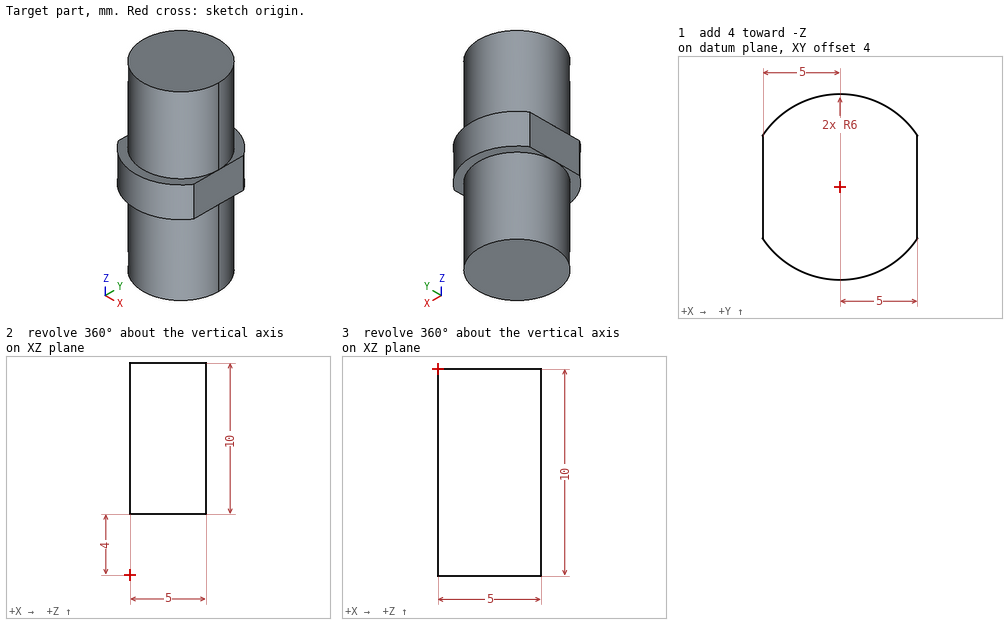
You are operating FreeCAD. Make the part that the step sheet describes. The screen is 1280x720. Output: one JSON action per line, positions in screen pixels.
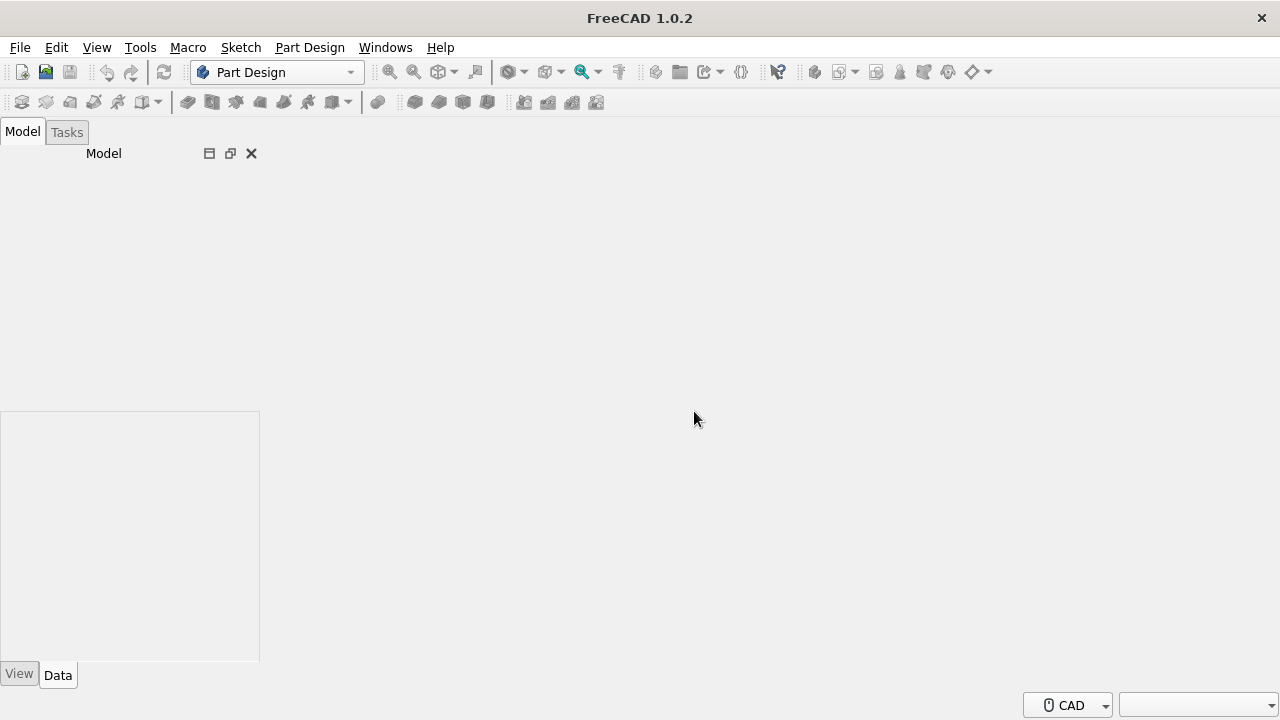
{"action": "left_click", "coordinate": [22, 72]}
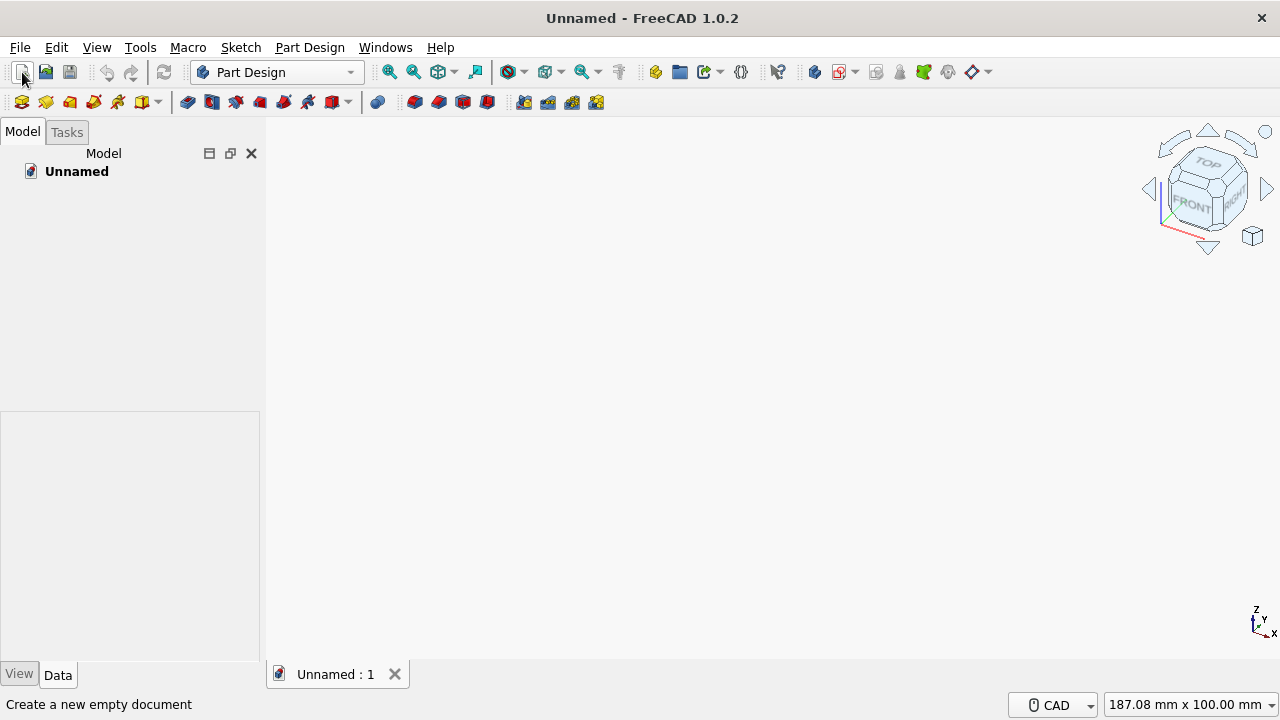
{"action": "left_click", "coordinate": [816, 72]}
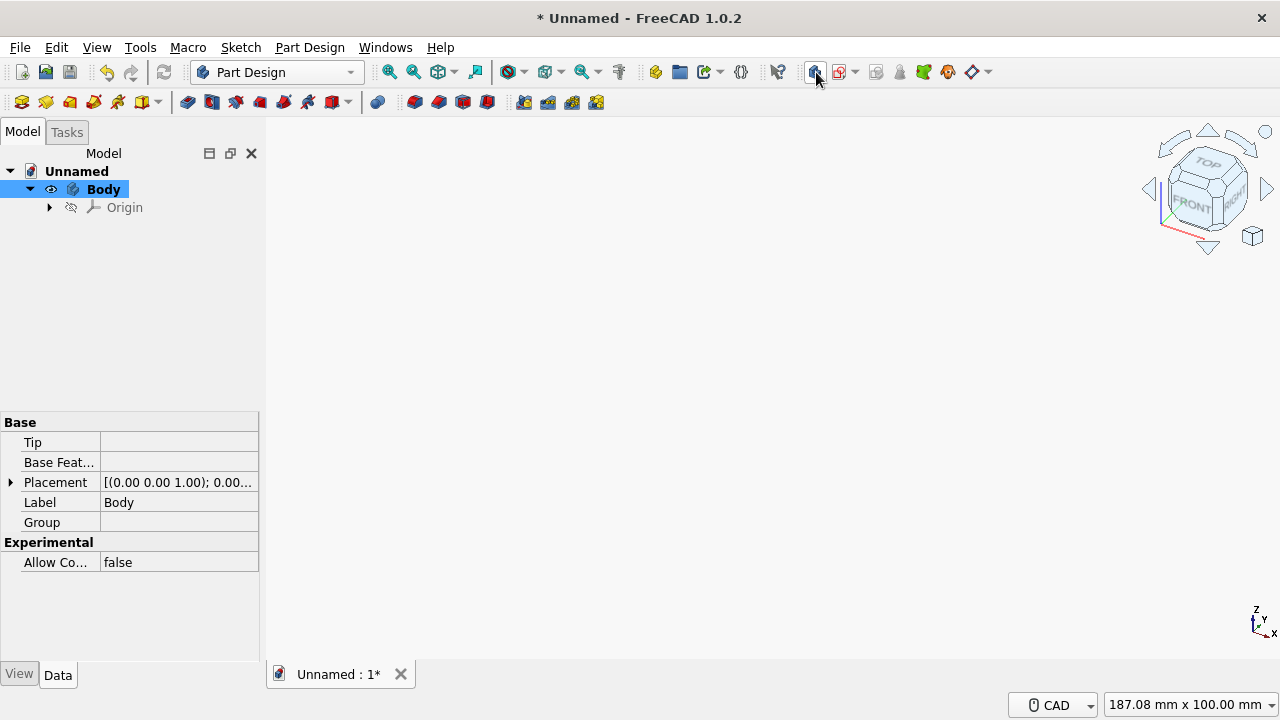
{"action": "left_click", "coordinate": [50, 207]}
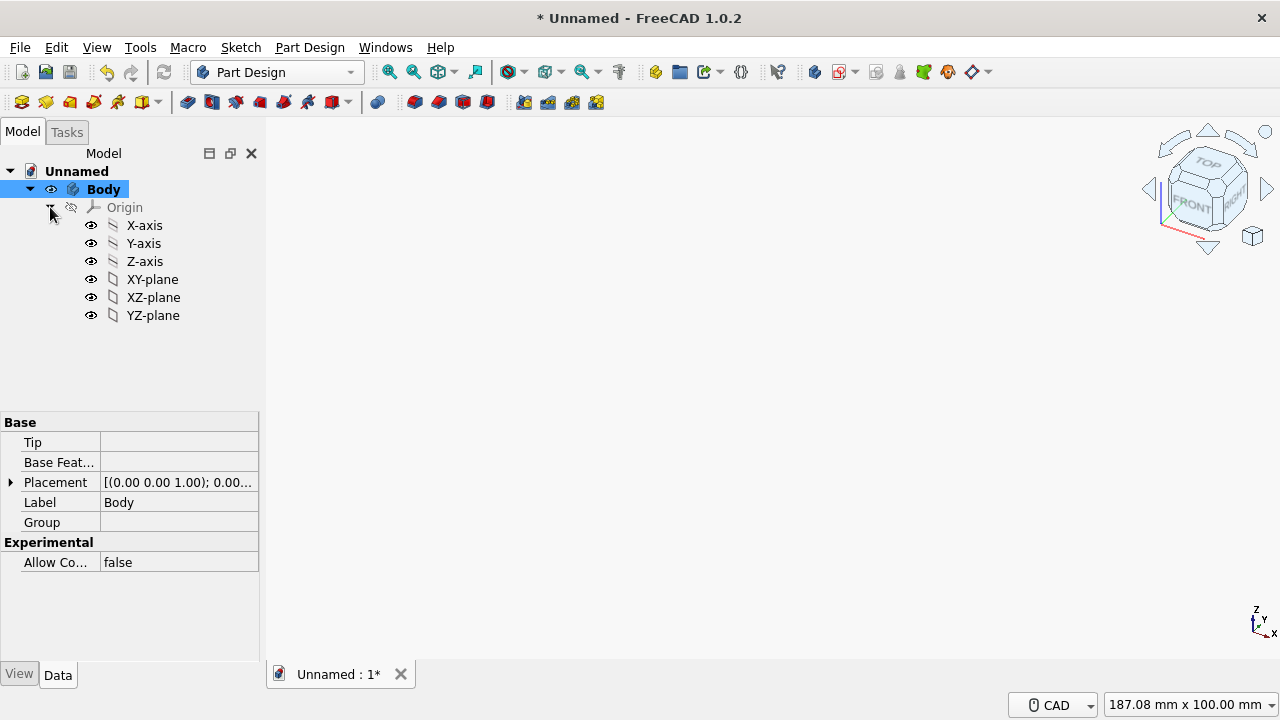
{"action": "left_click", "coordinate": [136, 279]}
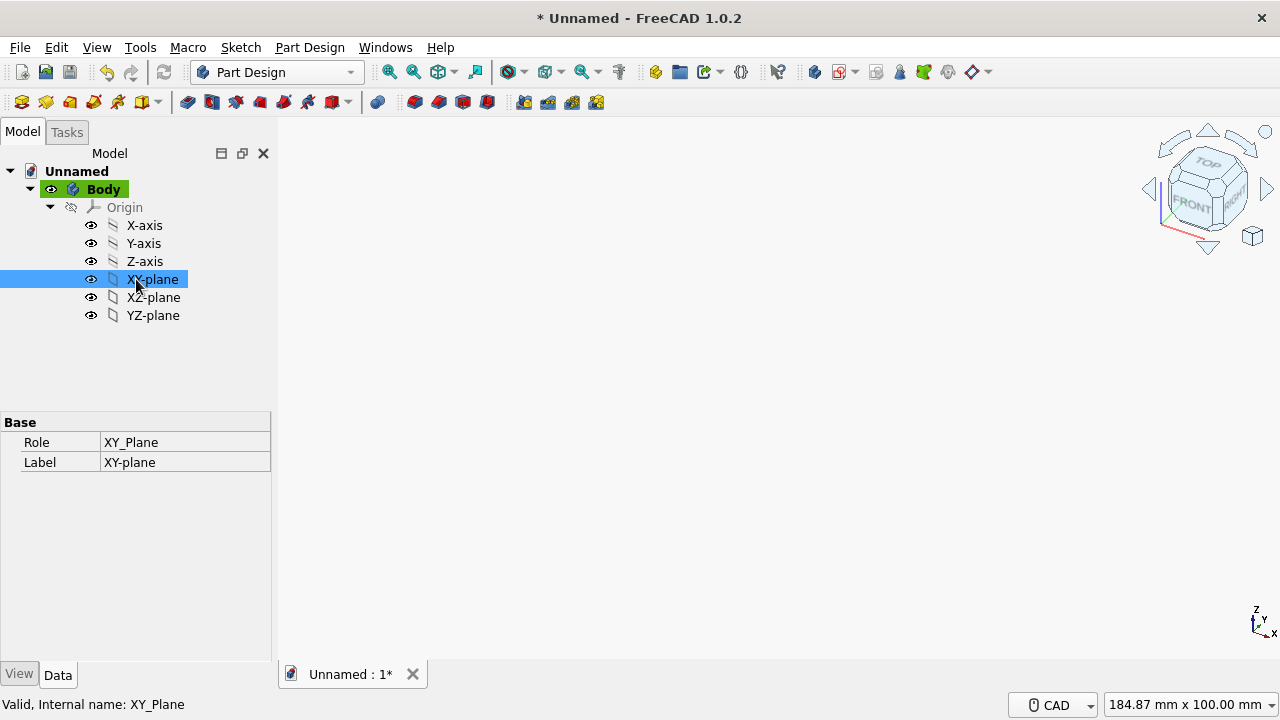
{"action": "left_click", "coordinate": [972, 72]}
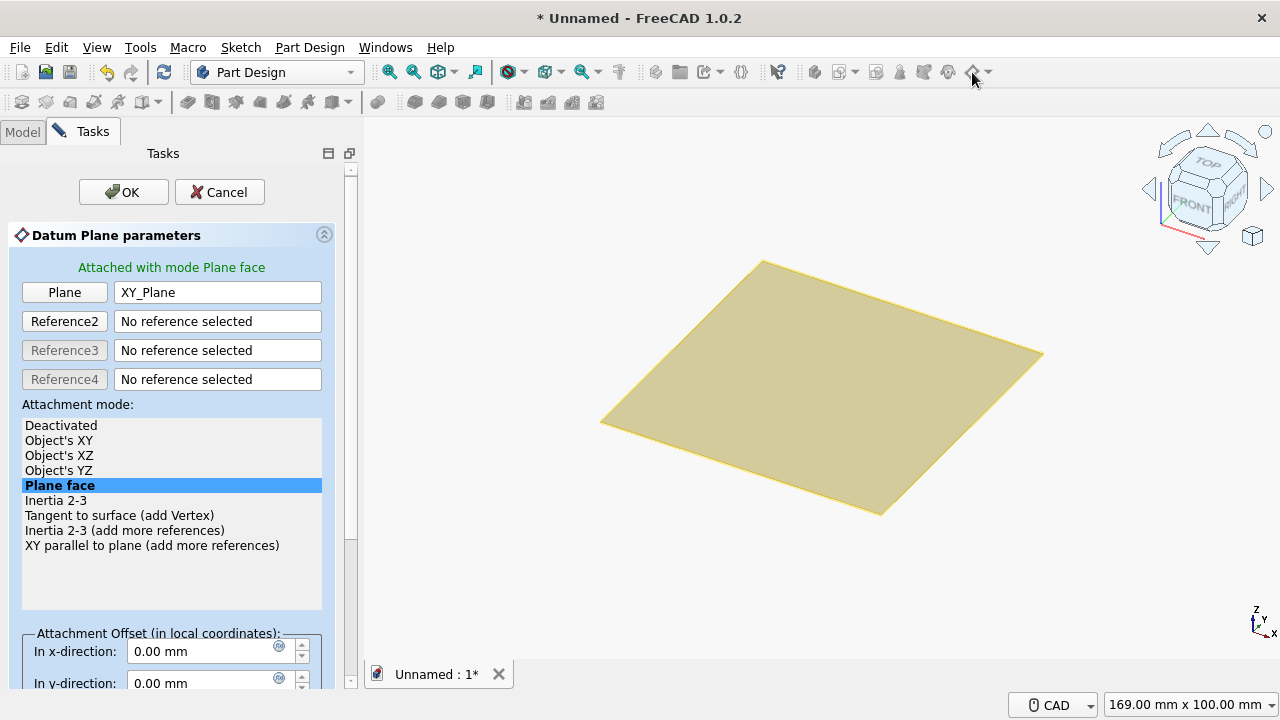
{"action": "scroll", "coordinate": [351, 426], "scroll_direction": "down", "scroll_amount": 2}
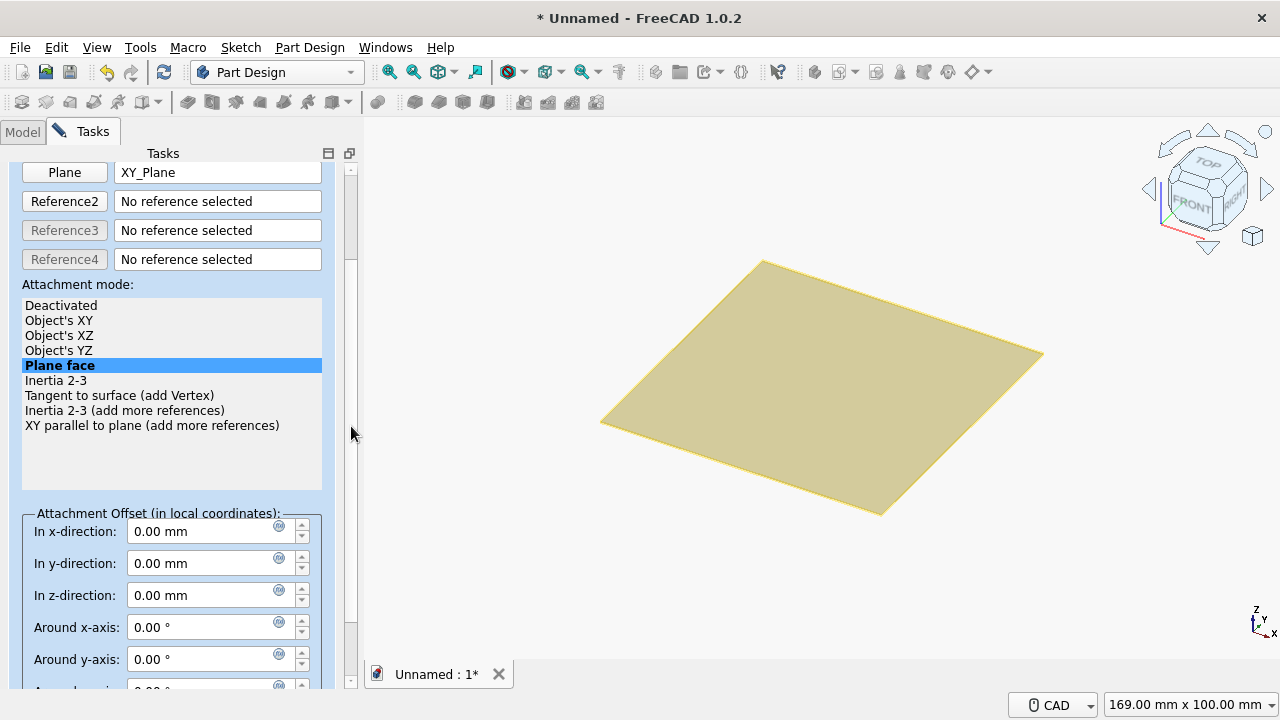
{"action": "triple_click", "coordinate": [210, 595]}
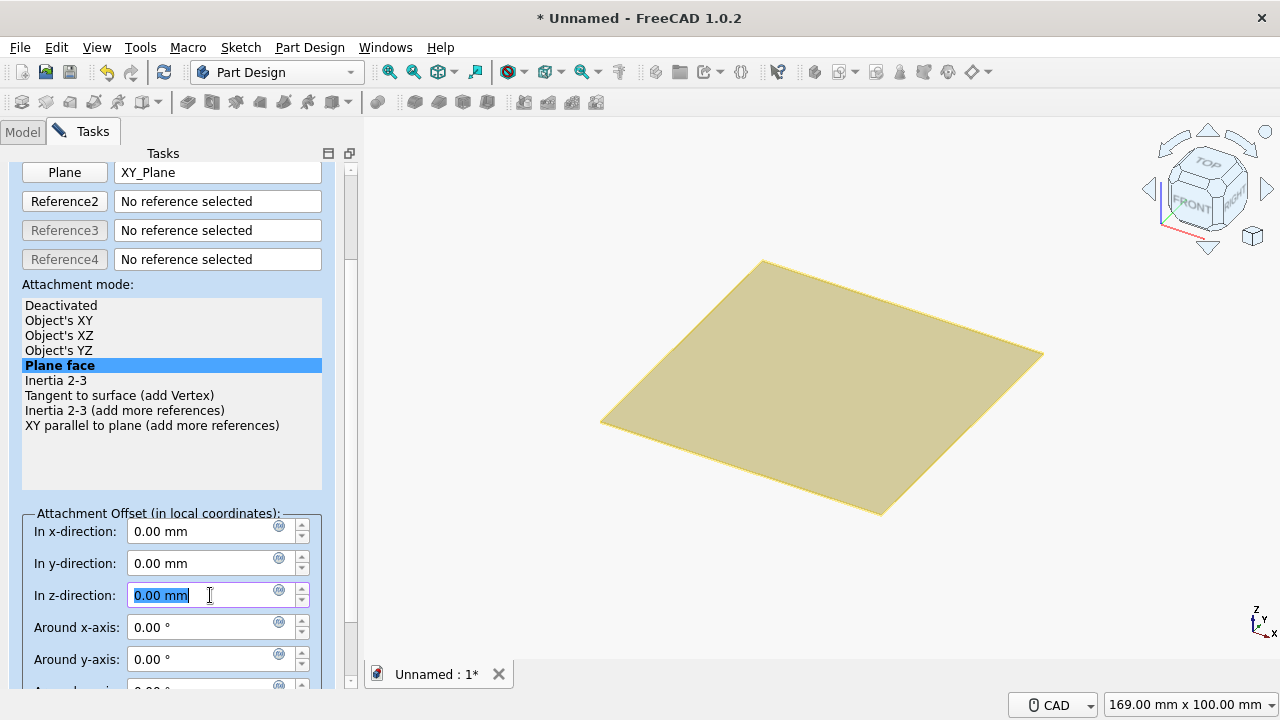
{"action": "type", "text": "4"}
{"action": "key", "text": "Tab"}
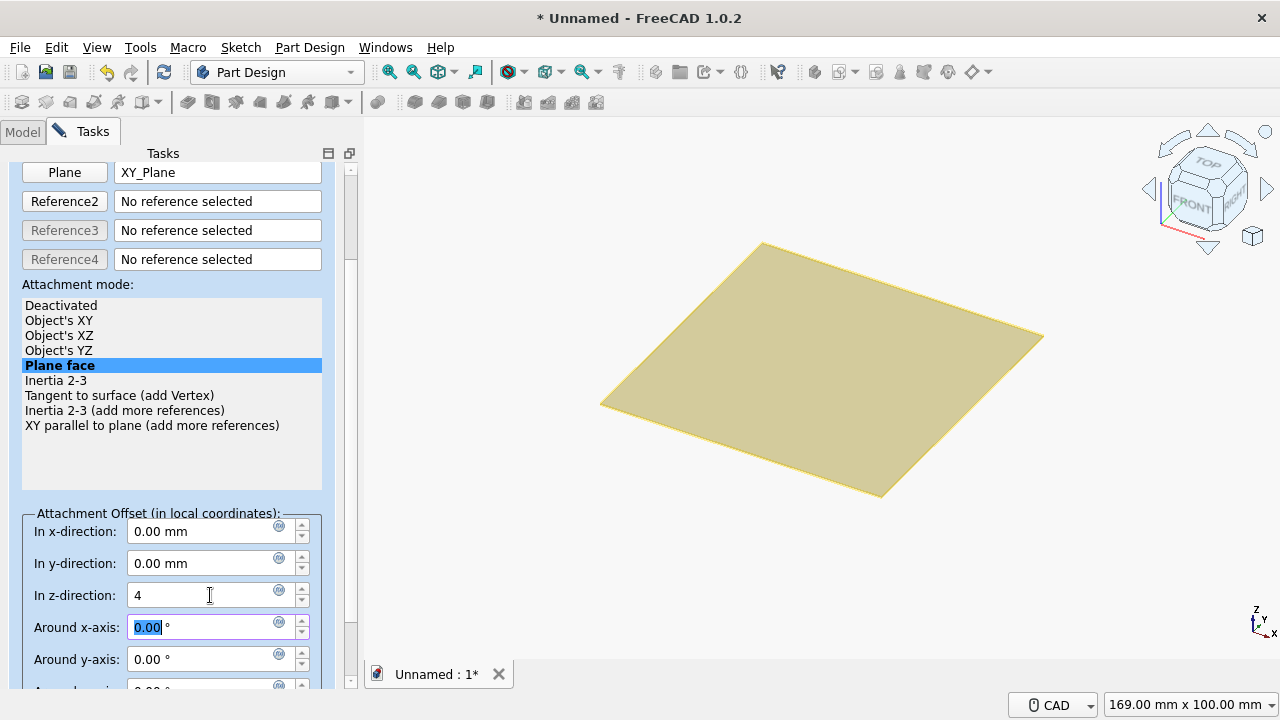
{"action": "scroll", "coordinate": [351, 426], "scroll_direction": "up", "scroll_amount": 3}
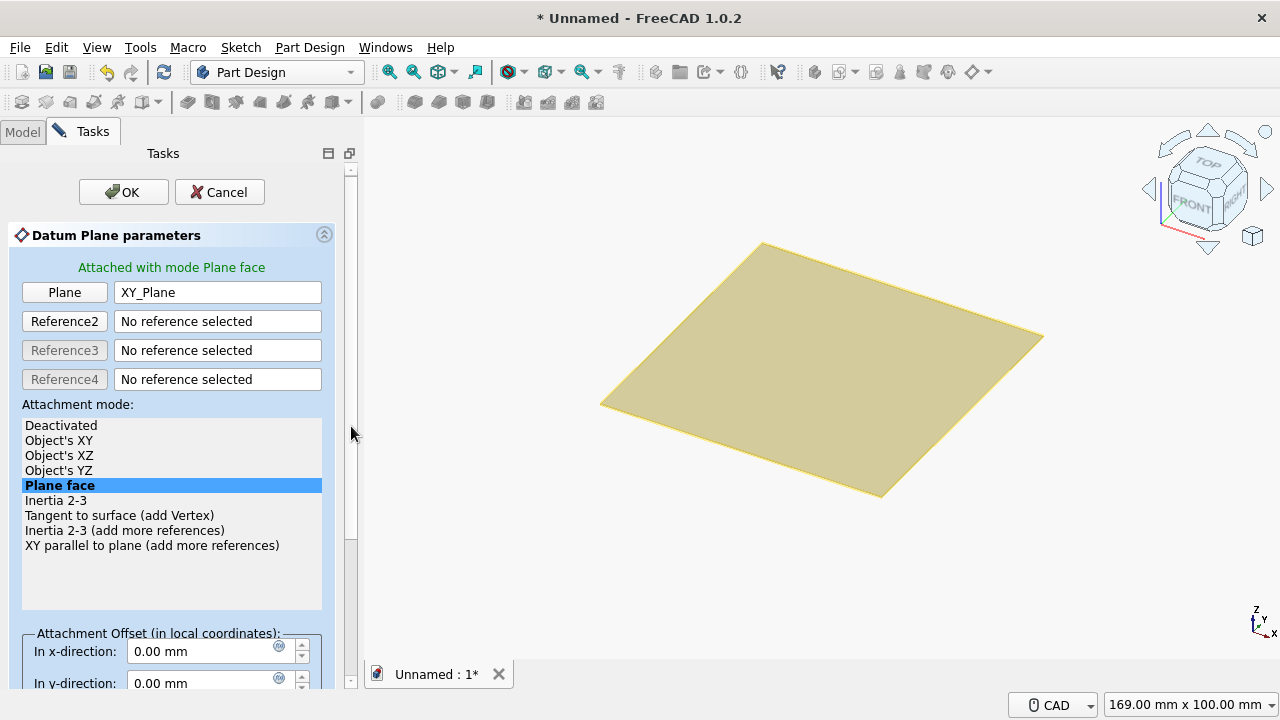
{"action": "left_click", "coordinate": [124, 192]}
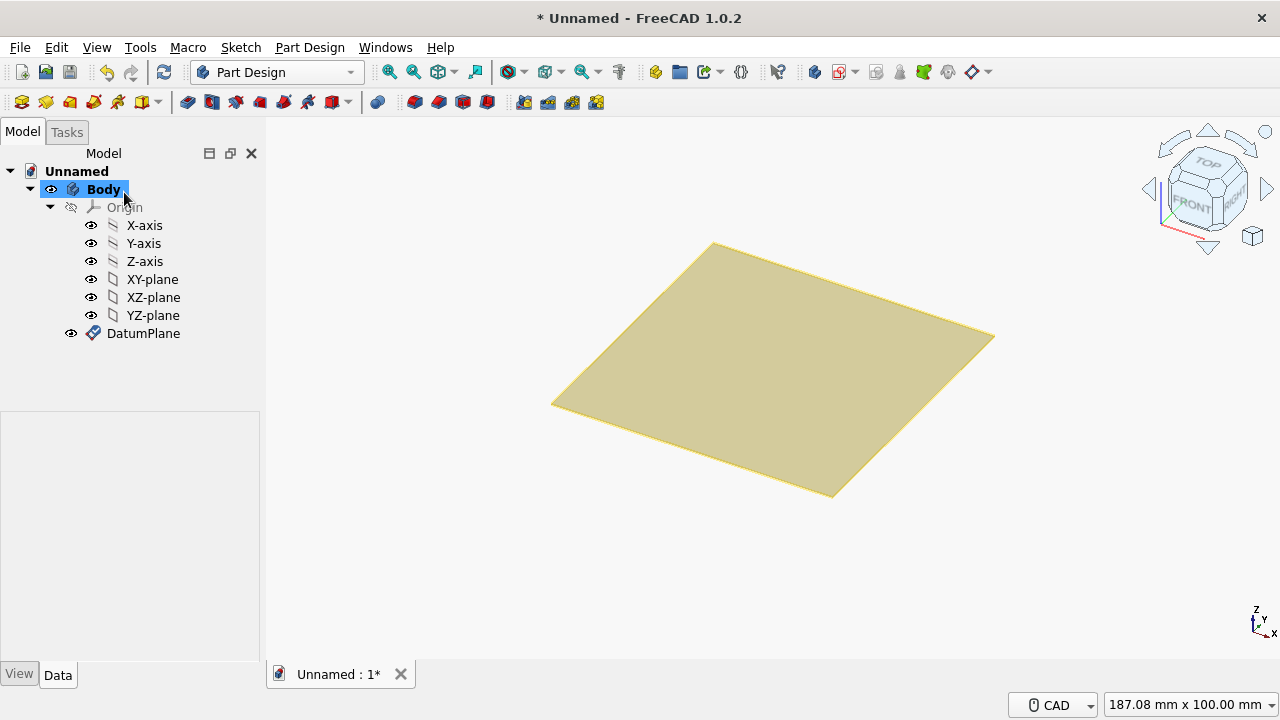
{"action": "left_click", "coordinate": [116, 333]}